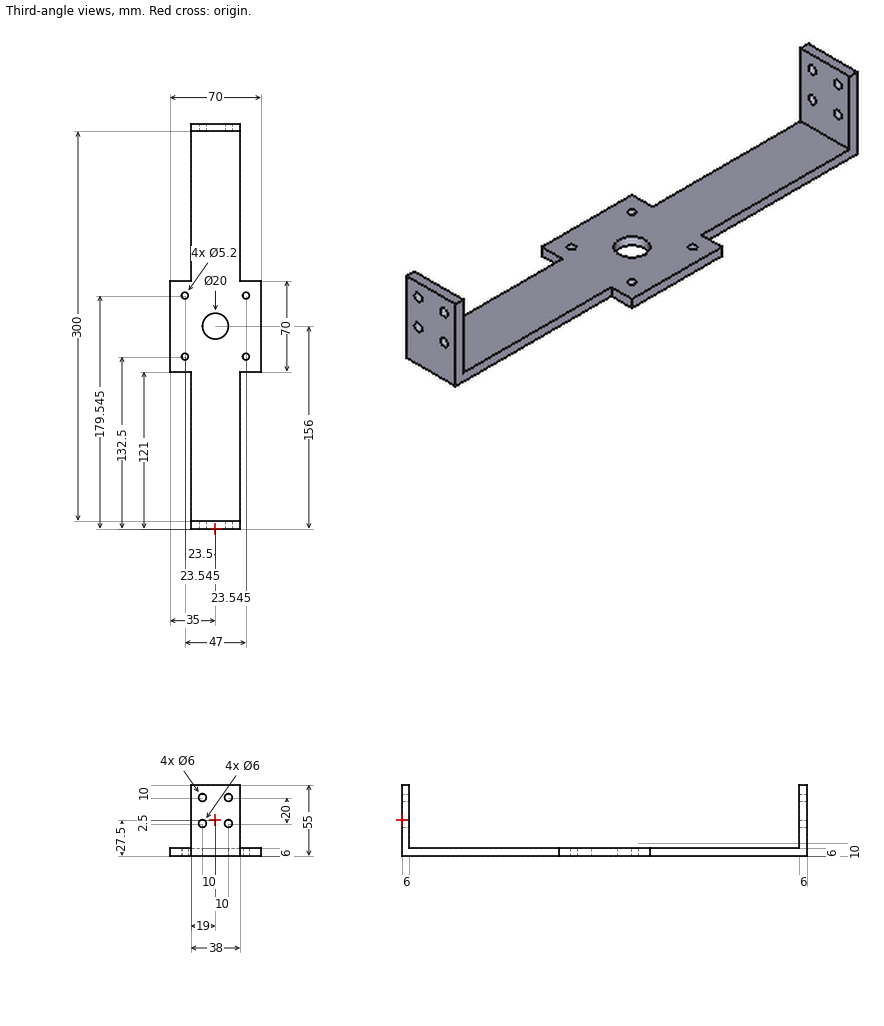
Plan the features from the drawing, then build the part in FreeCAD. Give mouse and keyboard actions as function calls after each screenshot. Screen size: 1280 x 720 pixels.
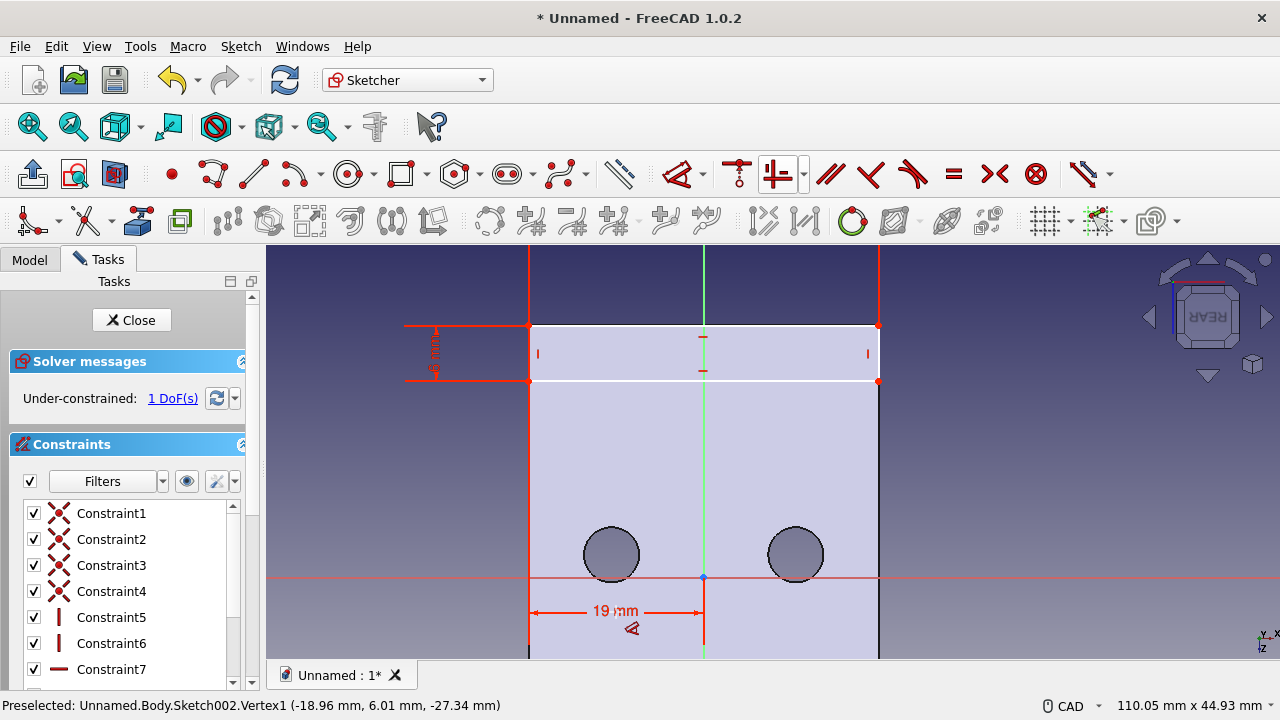
click(529, 326)
click(495, 452)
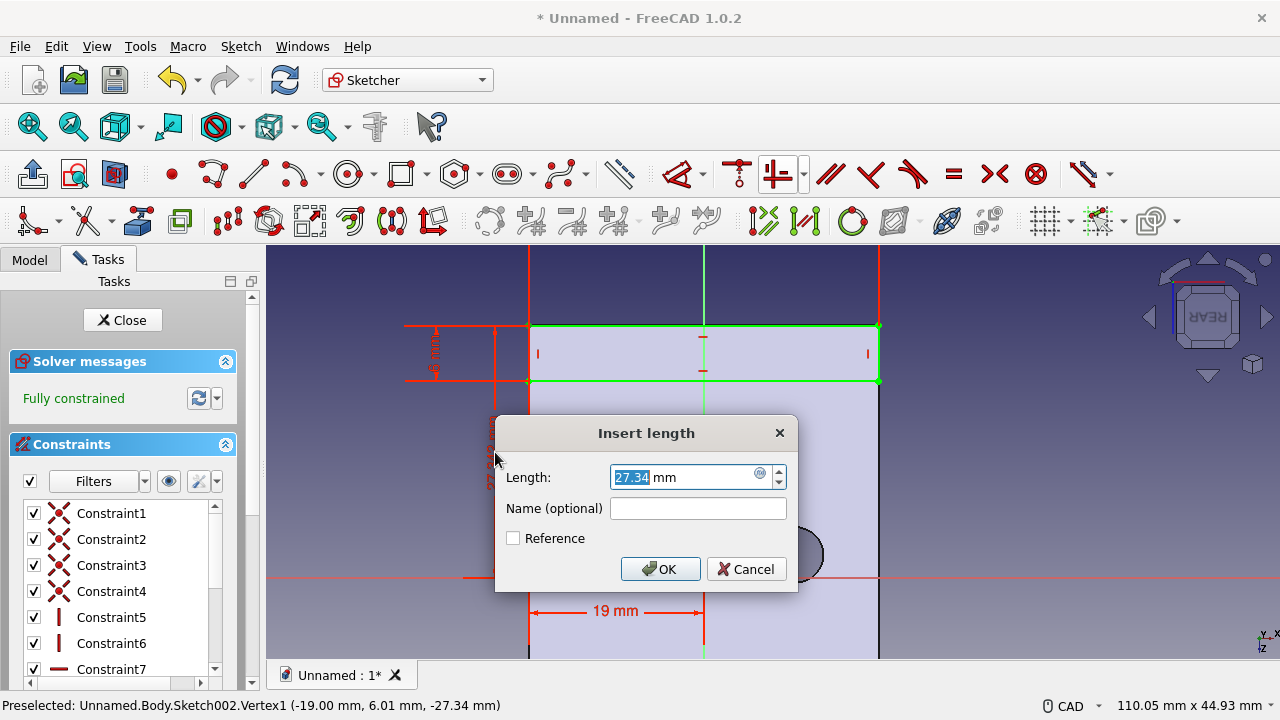
text(27.5)
key(Return)
key(Escape)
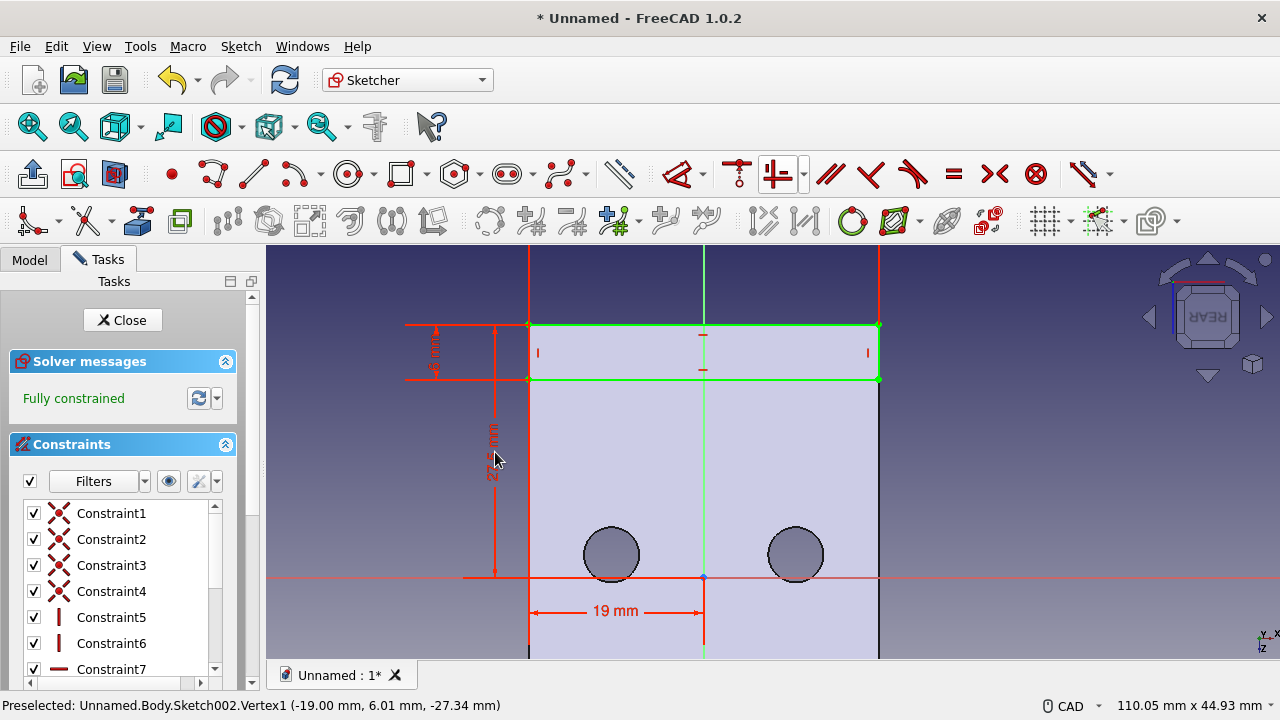
click(123, 320)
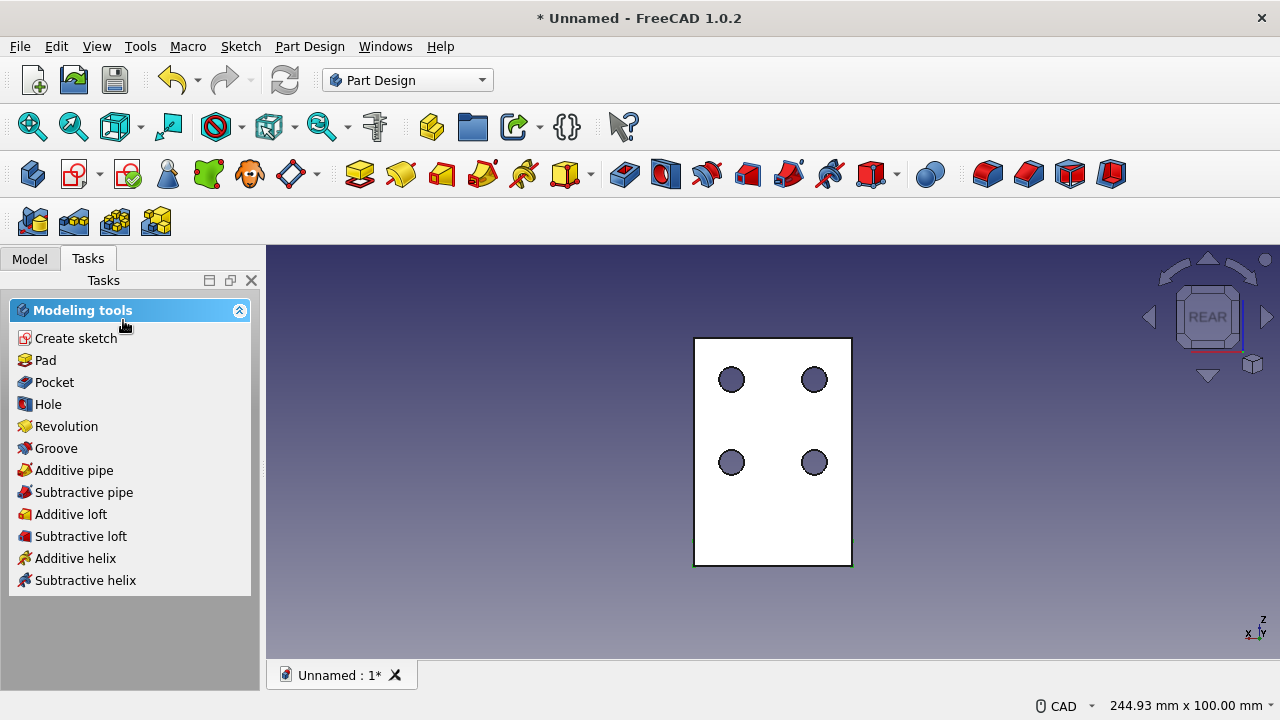
click(360, 174)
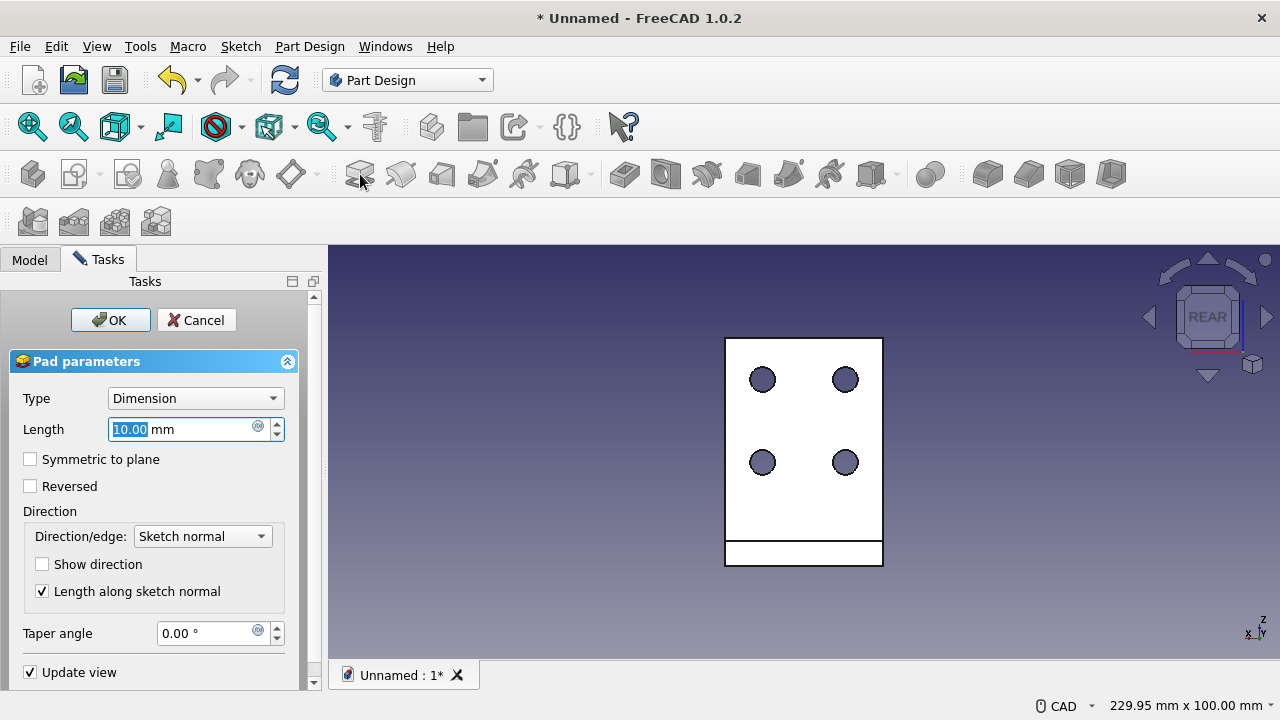
text(300)
key(Tab)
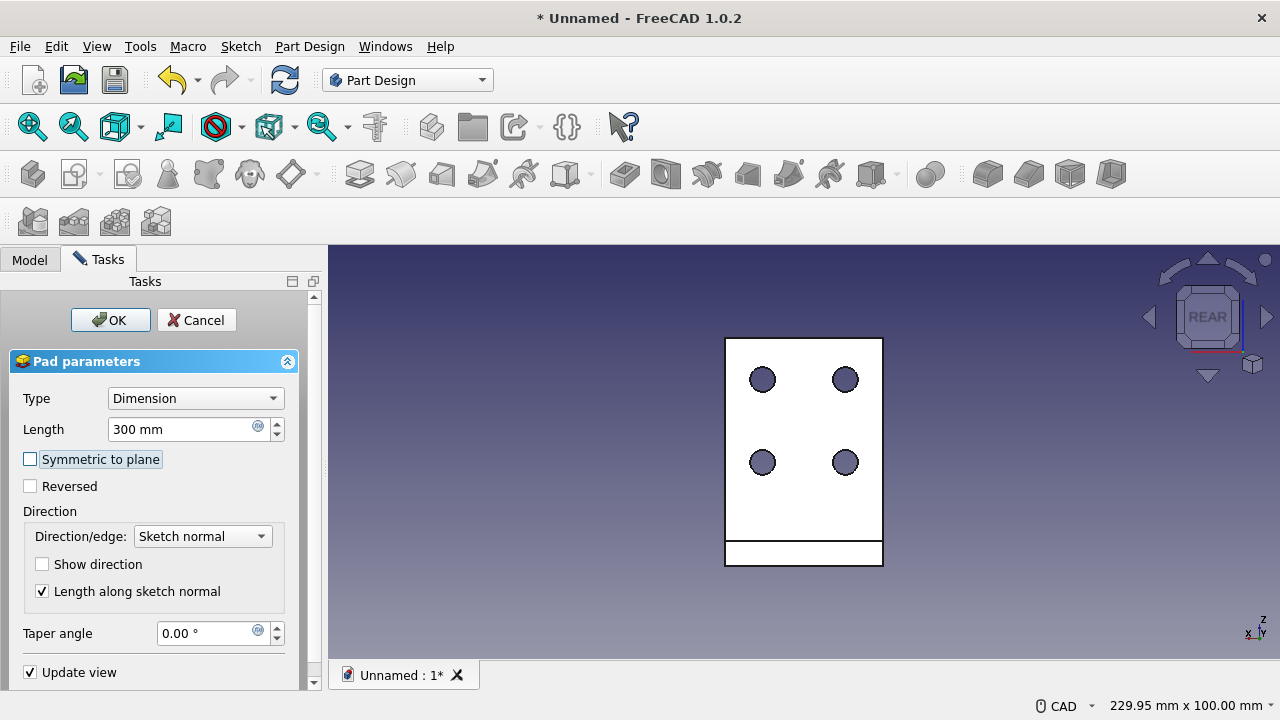
click(111, 320)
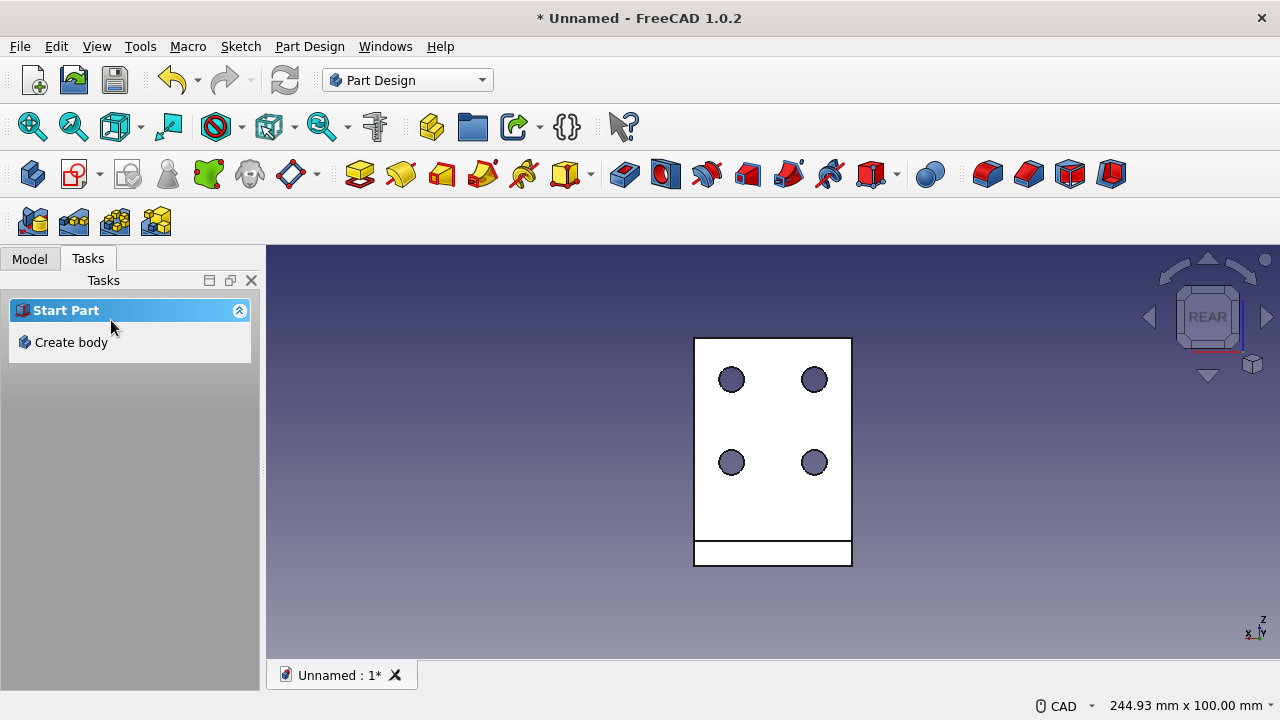
click(30, 258)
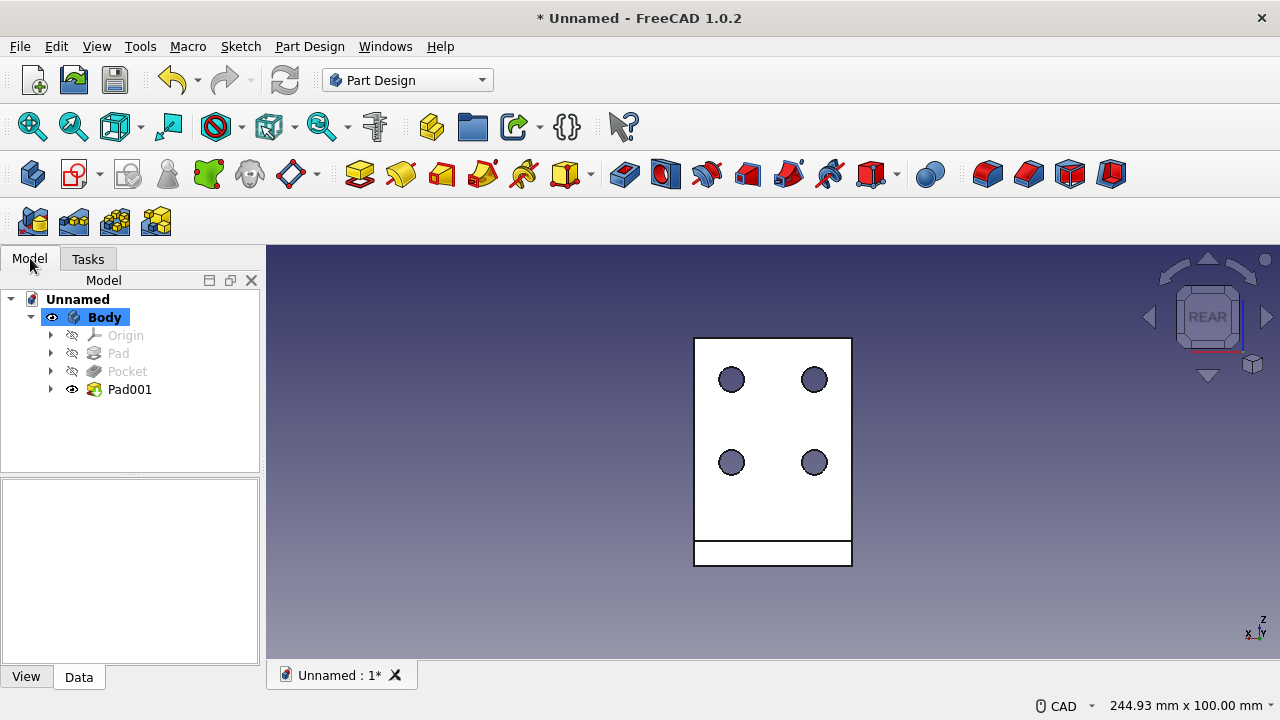
click(51, 335)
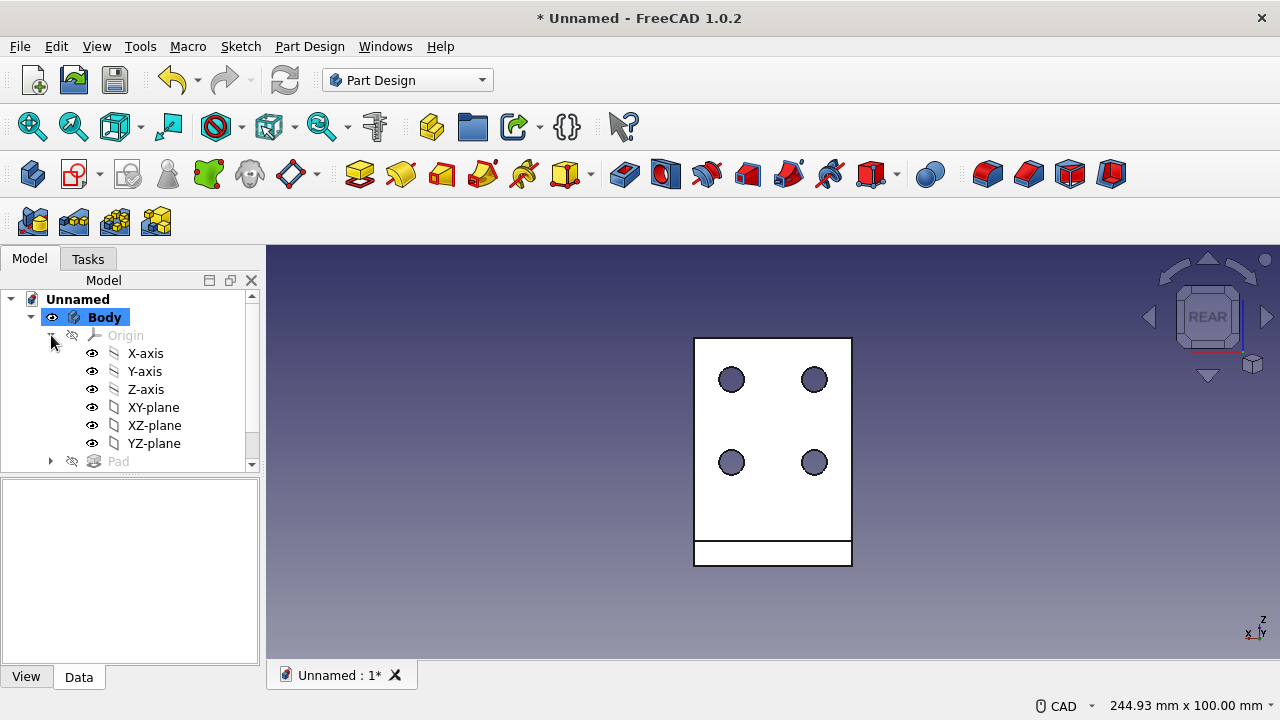
click(137, 425)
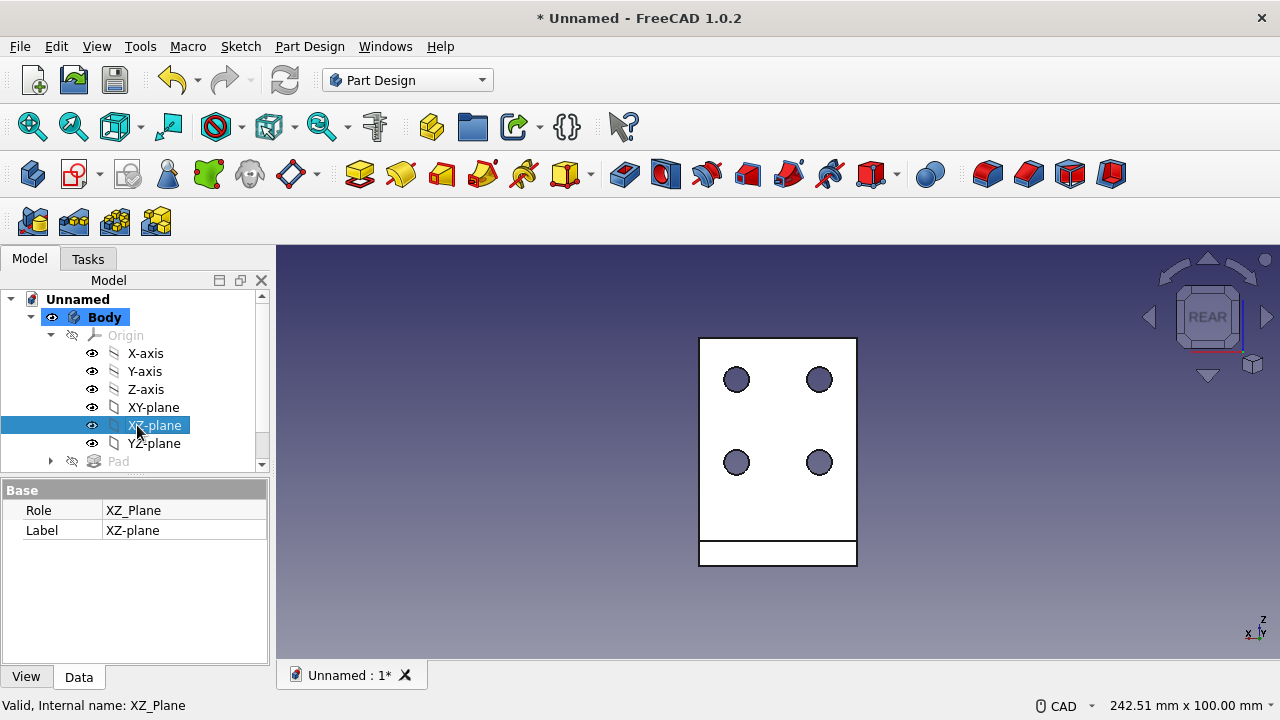
click(290, 174)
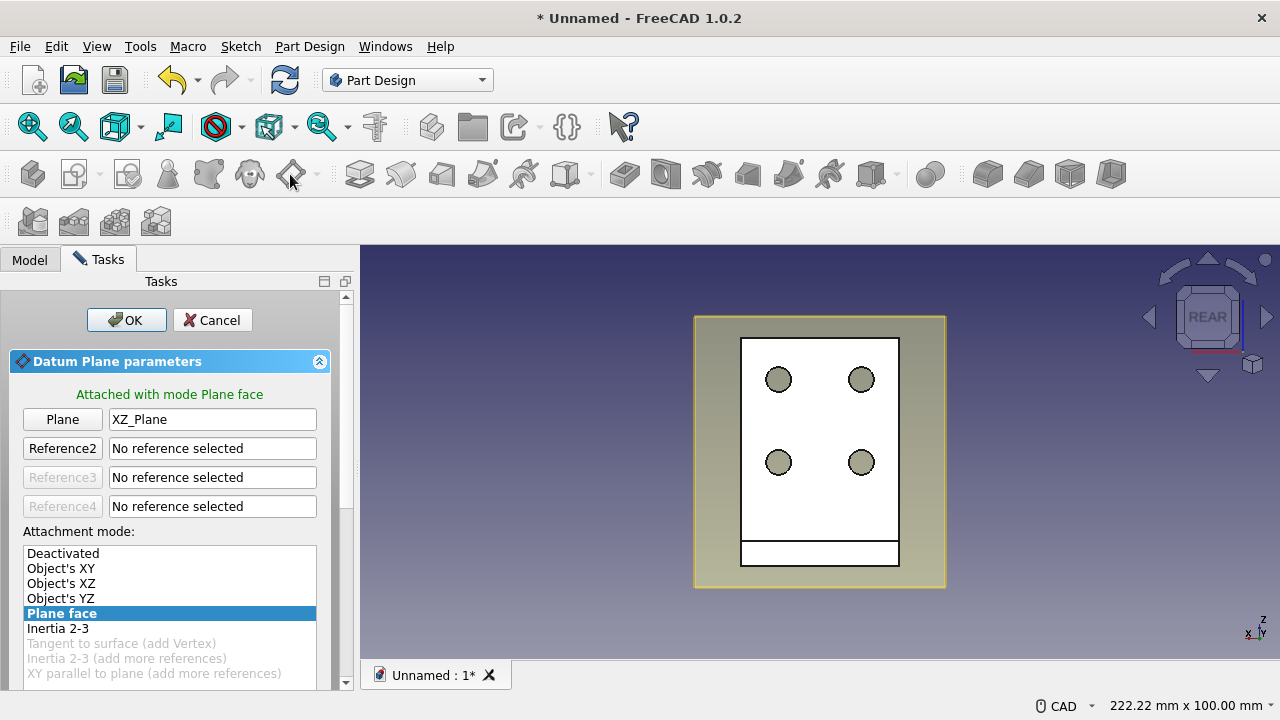
scroll(346, 490, down, 4)